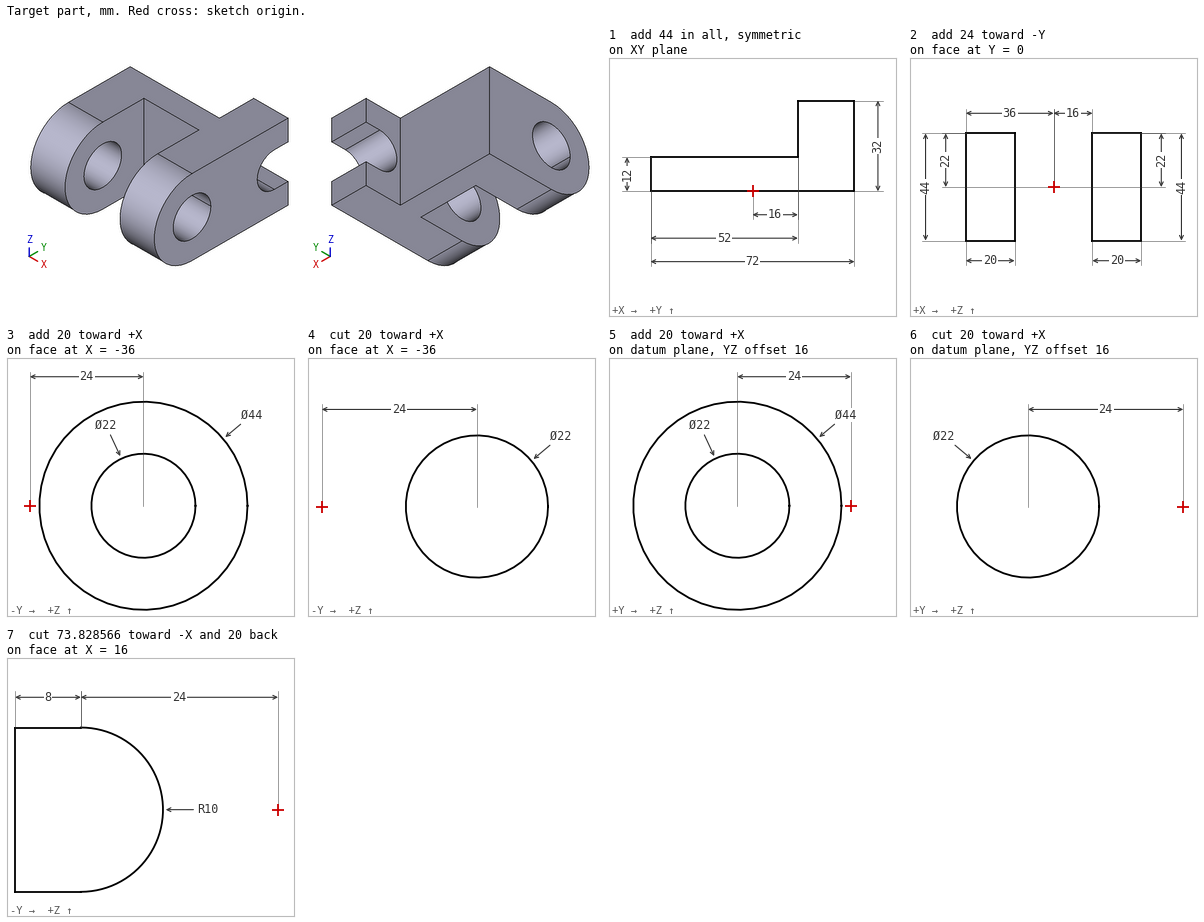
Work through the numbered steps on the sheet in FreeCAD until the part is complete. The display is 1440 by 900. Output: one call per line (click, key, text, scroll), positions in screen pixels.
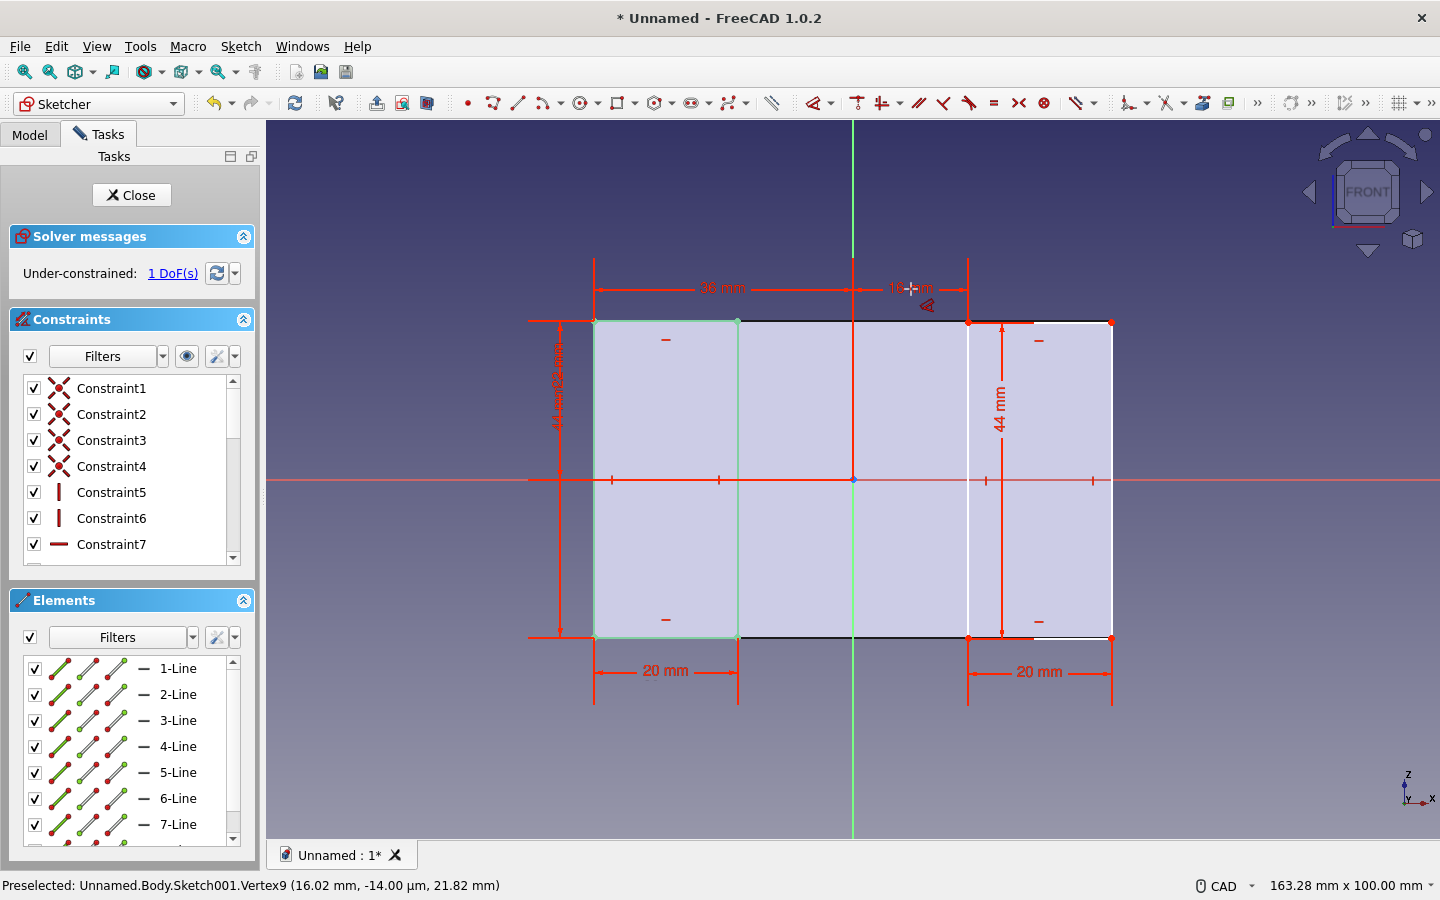
click(968, 323)
click(1002, 365)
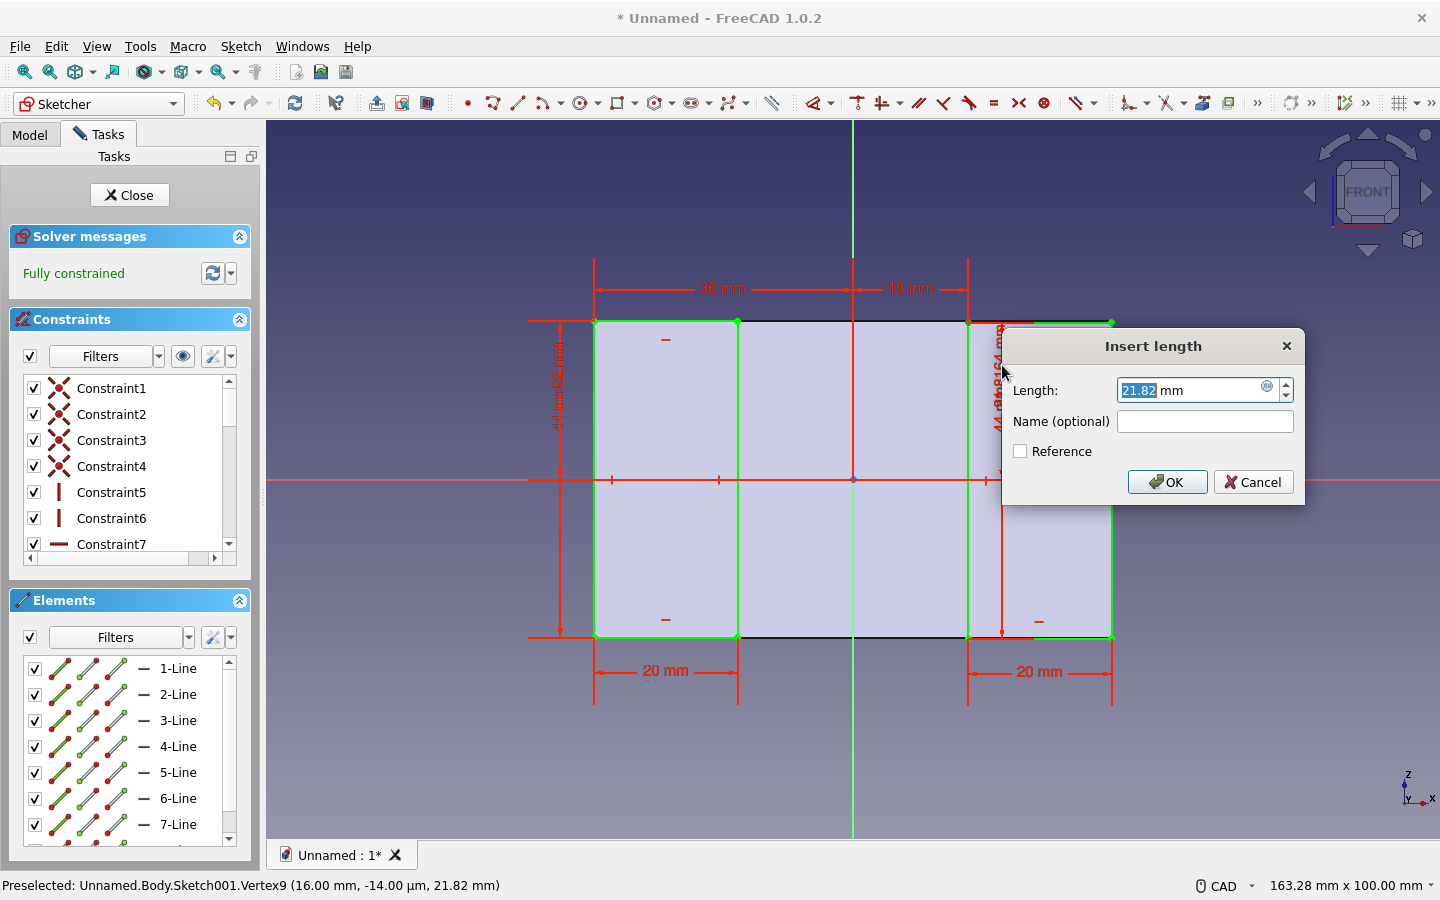
text(22)
key(Return)
key(Escape)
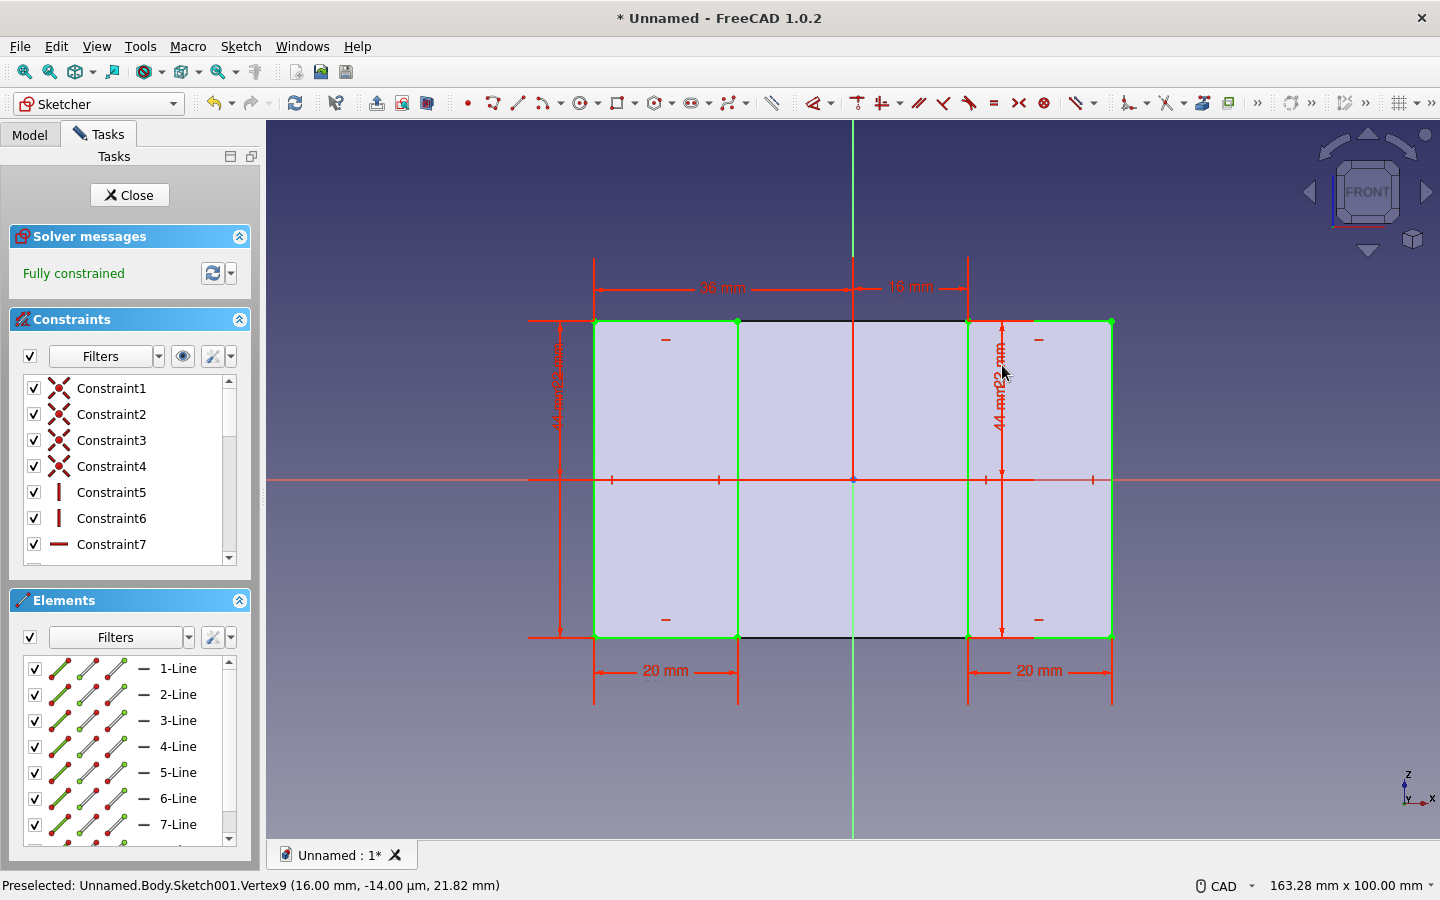
click(130, 195)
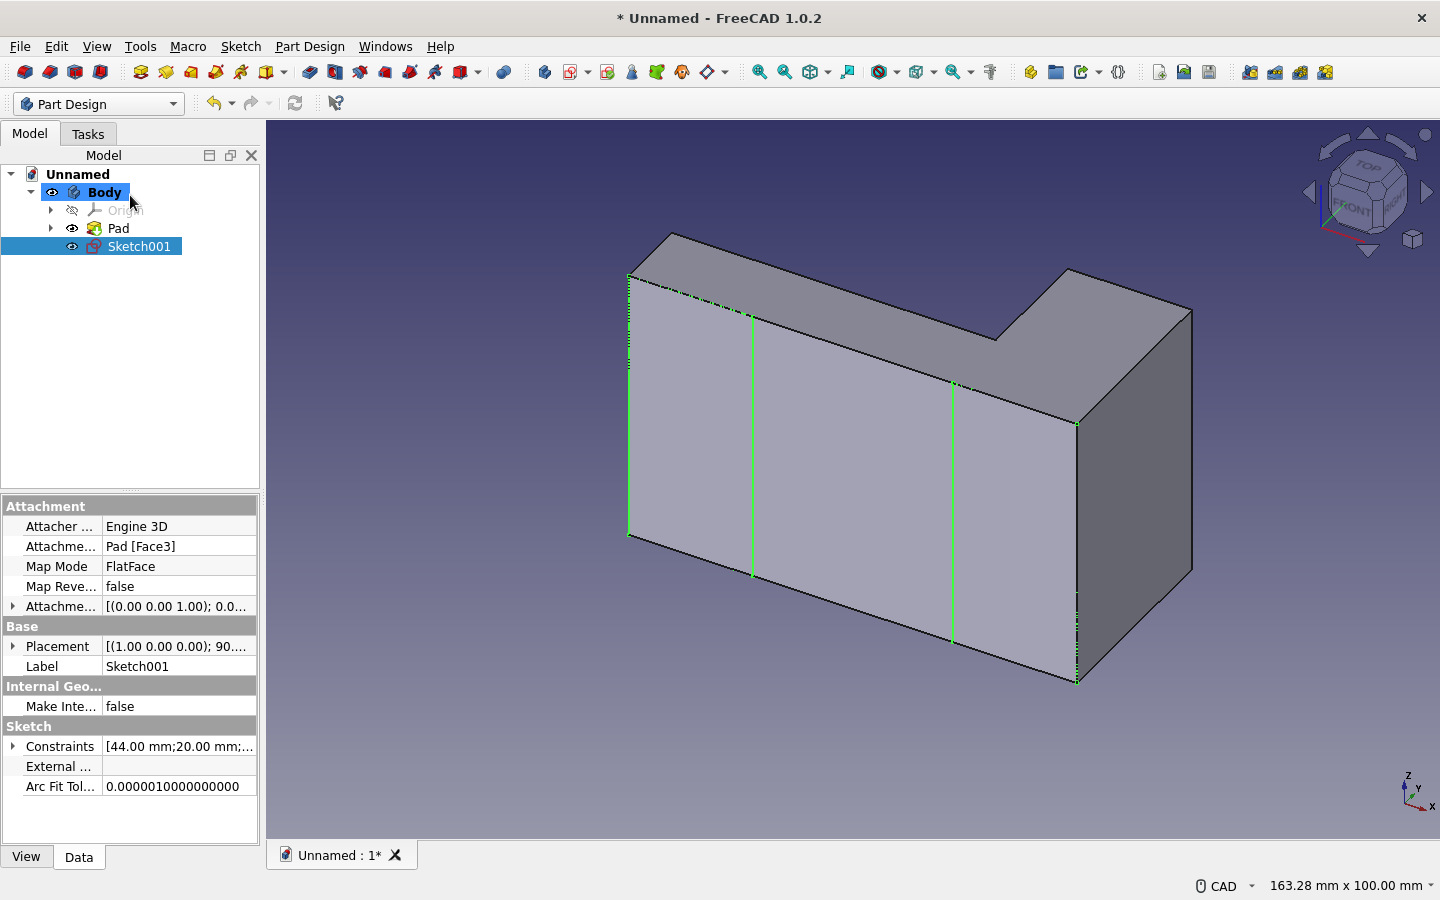
click(141, 72)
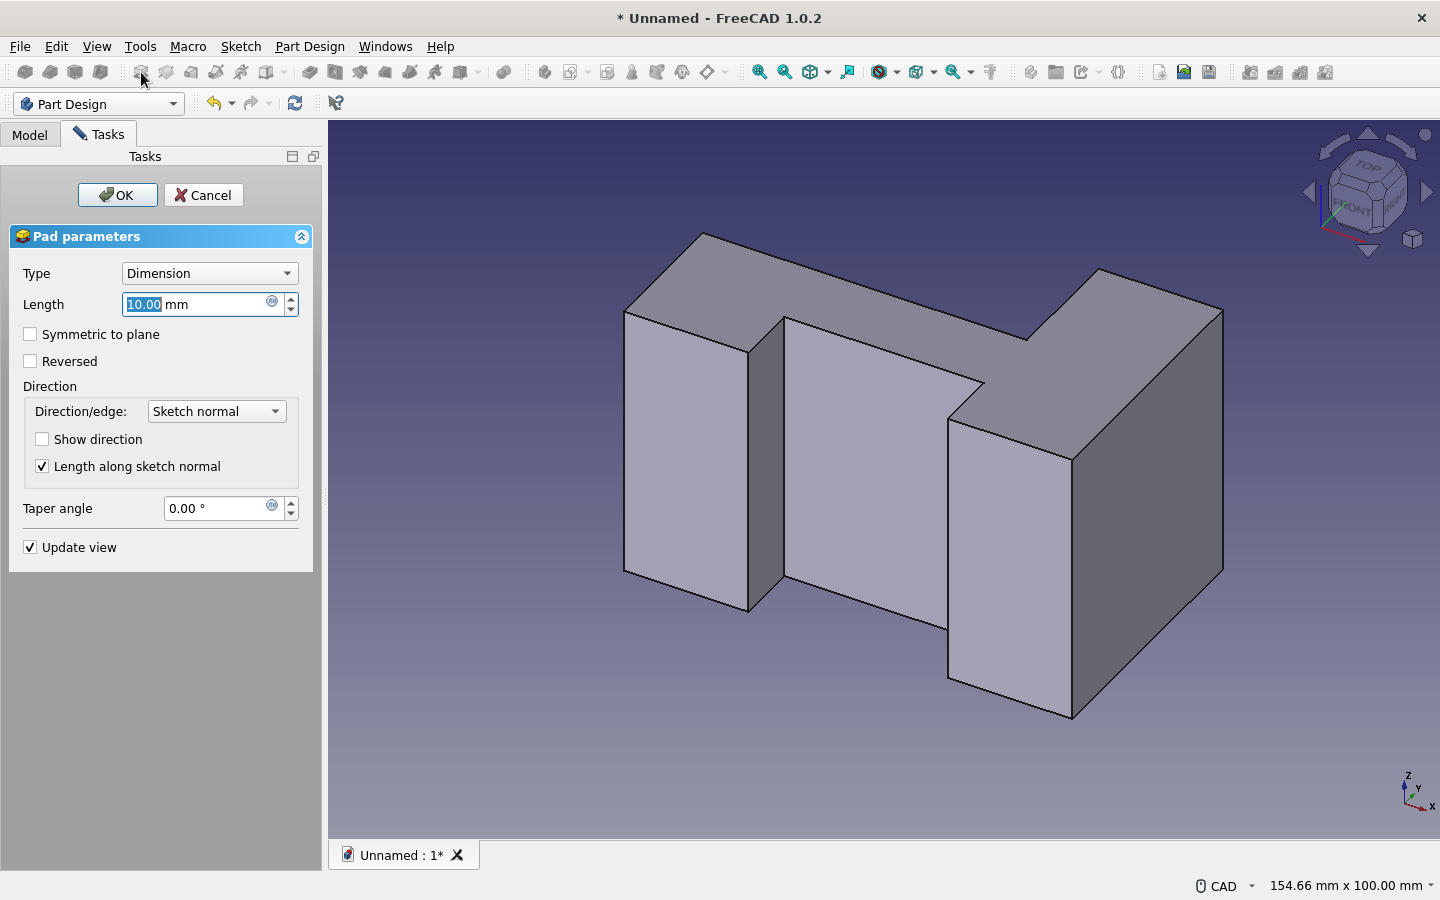
text(24)
key(Tab)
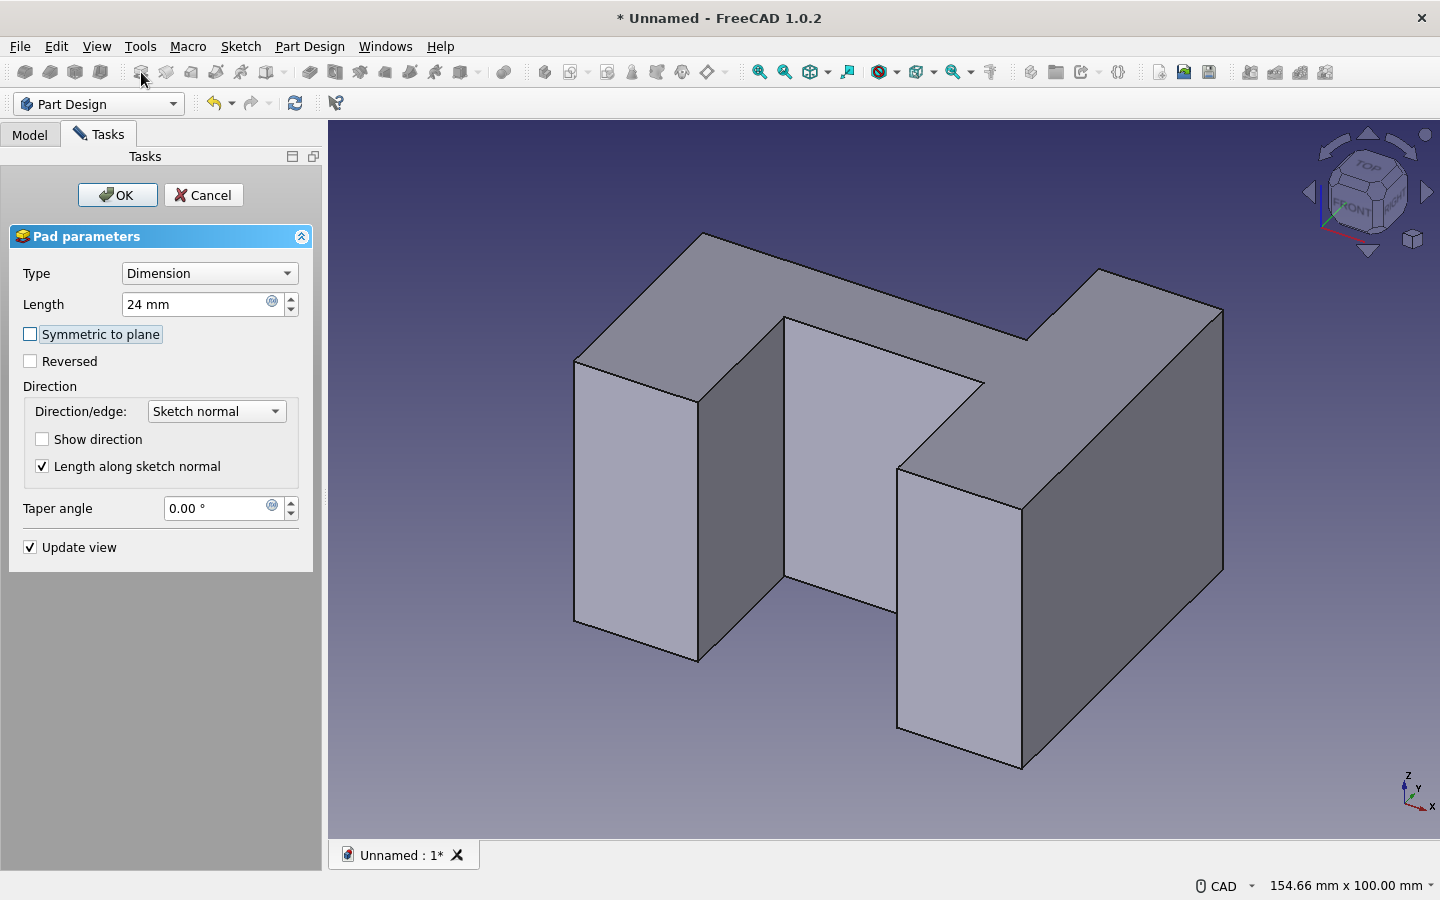
click(118, 195)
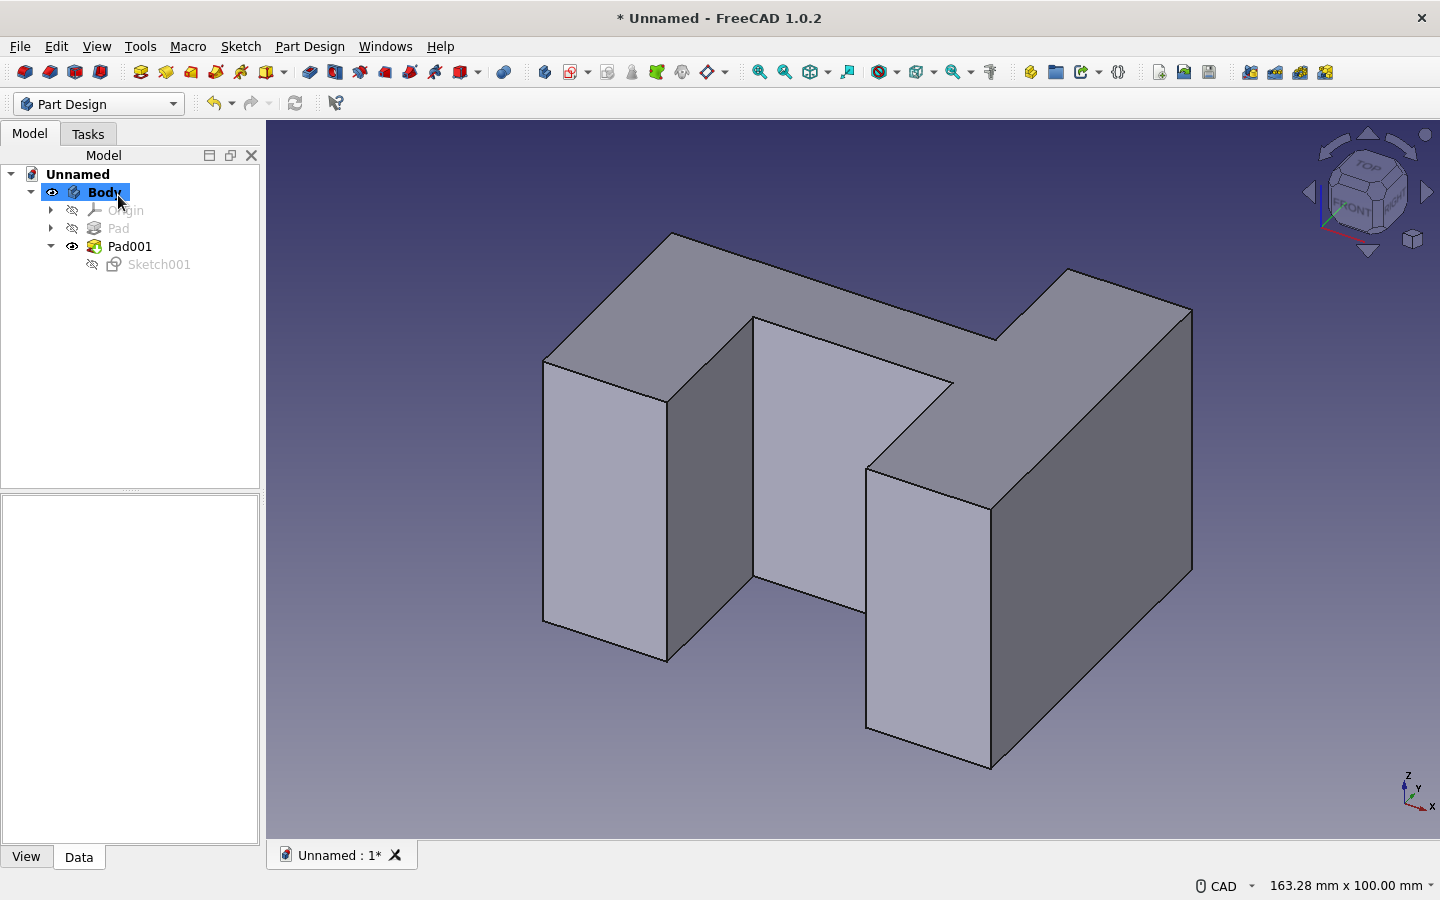
key(6)